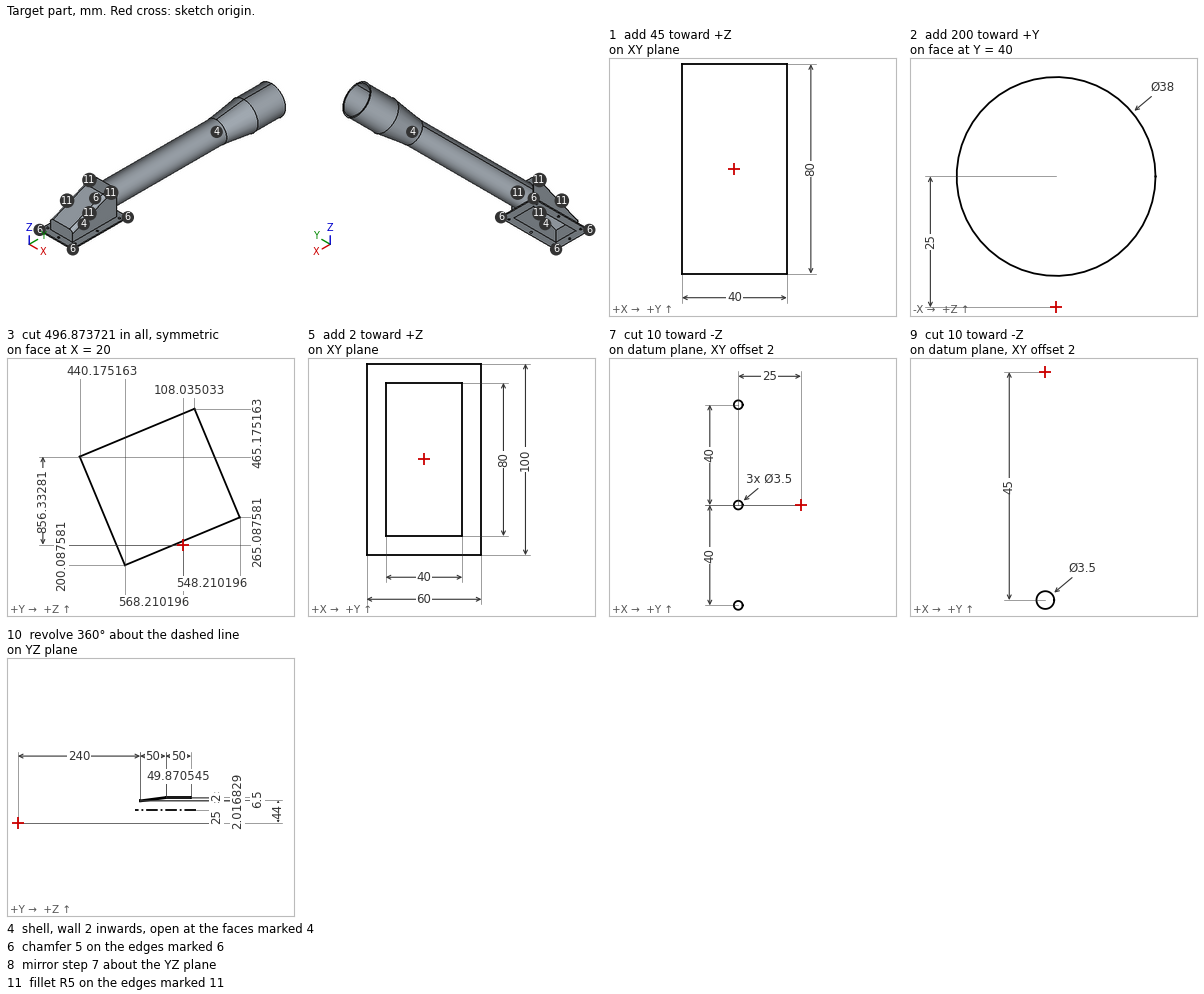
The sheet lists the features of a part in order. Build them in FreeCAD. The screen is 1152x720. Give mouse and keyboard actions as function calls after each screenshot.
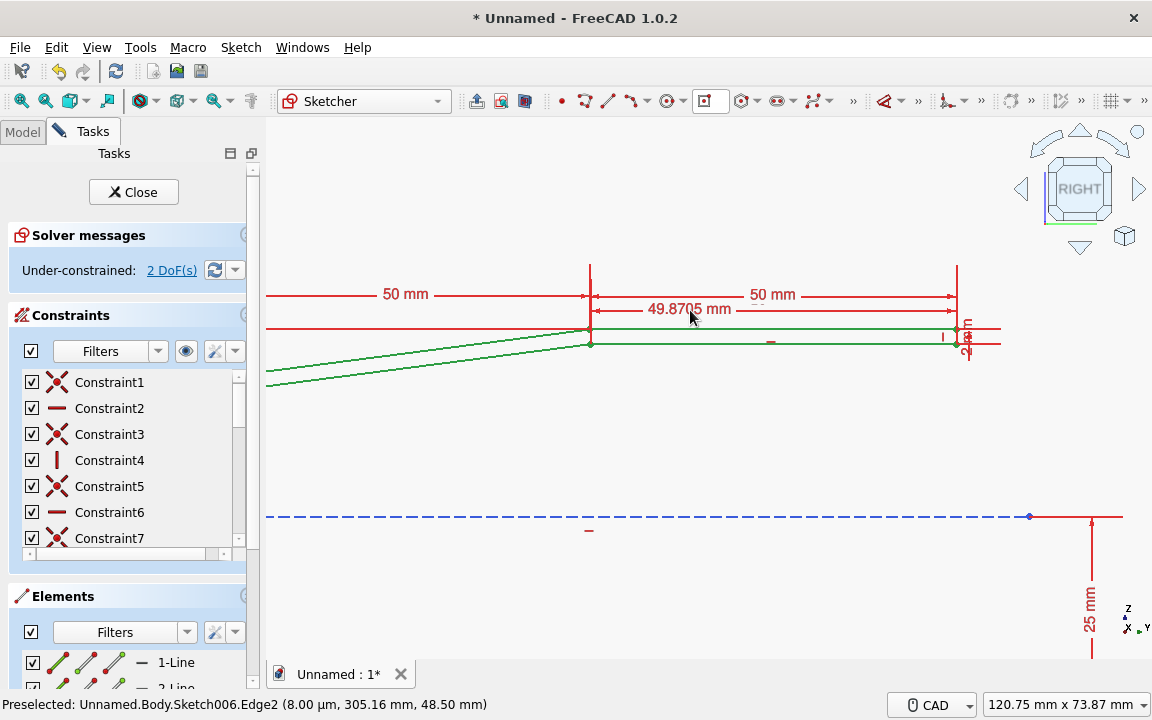
click(134, 192)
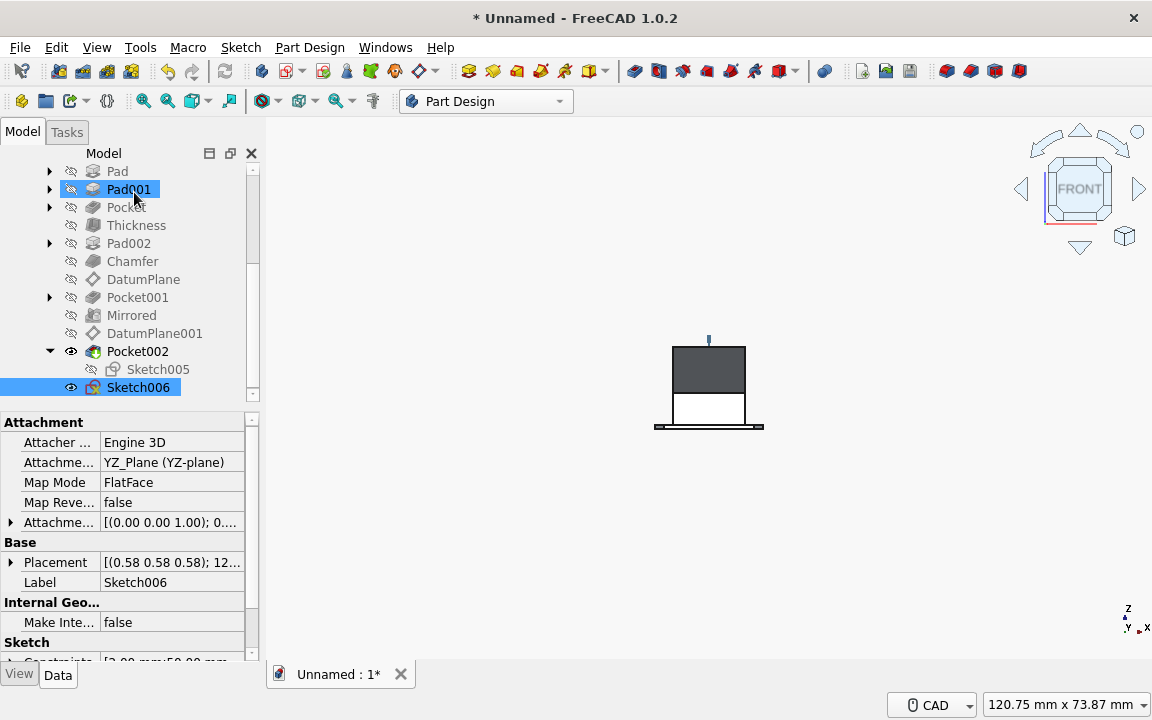
click(494, 72)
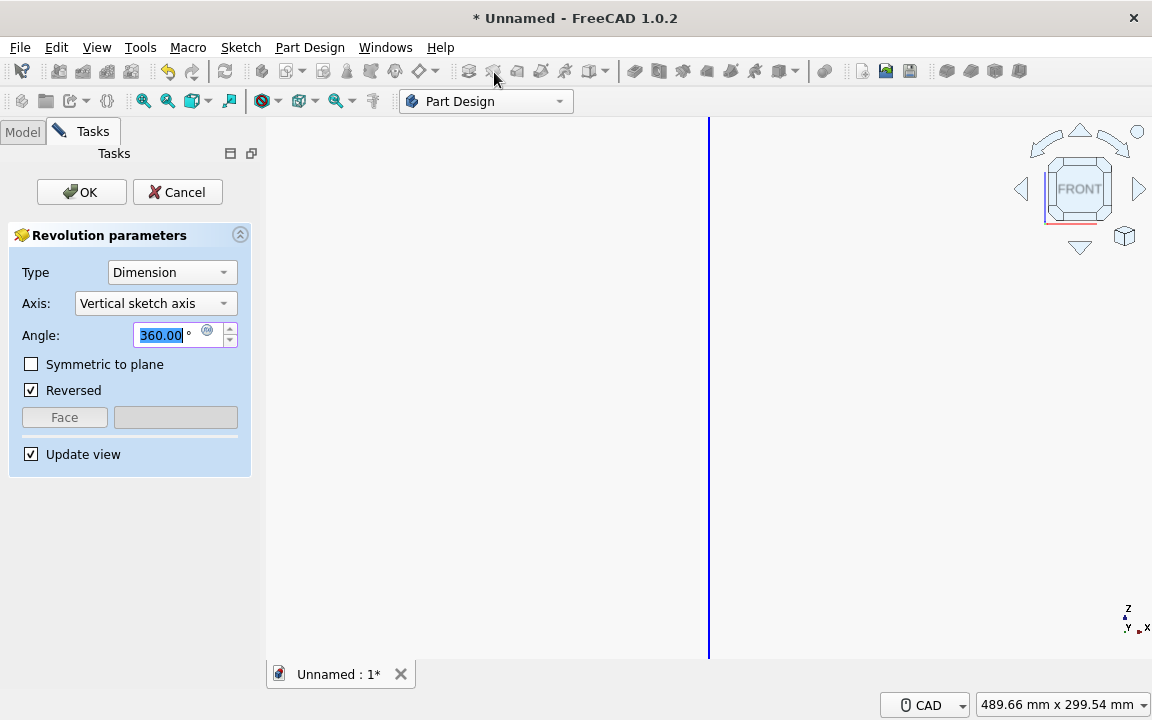
click(156, 304)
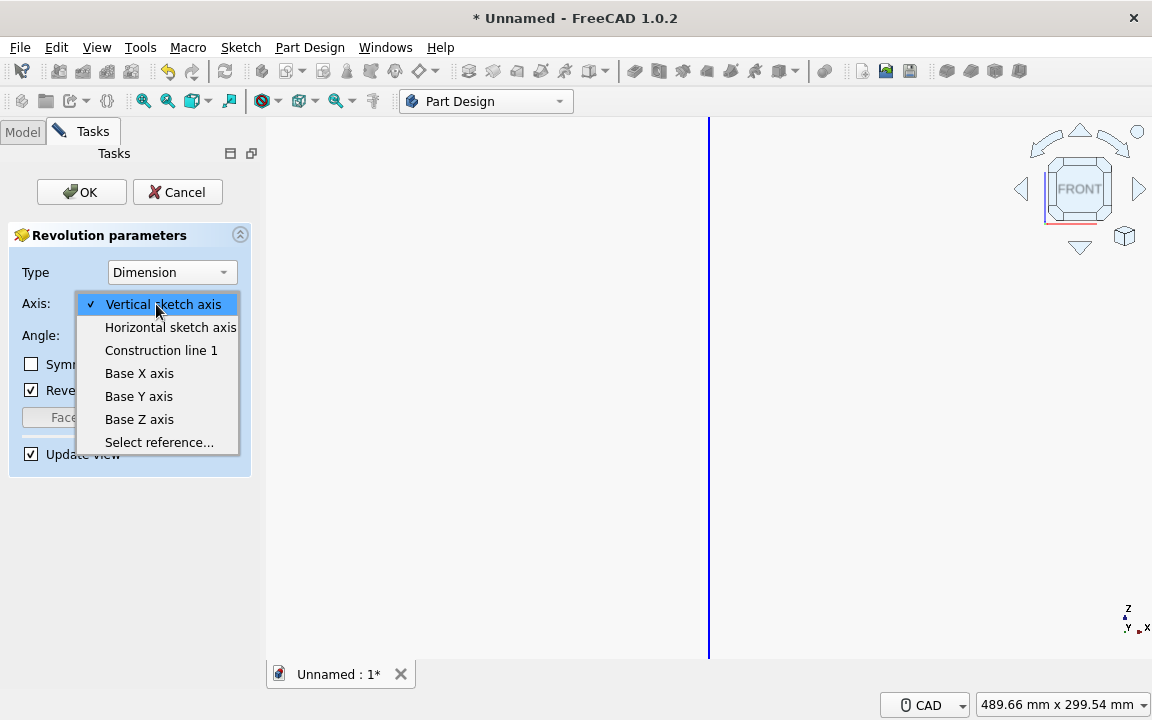
click(156, 350)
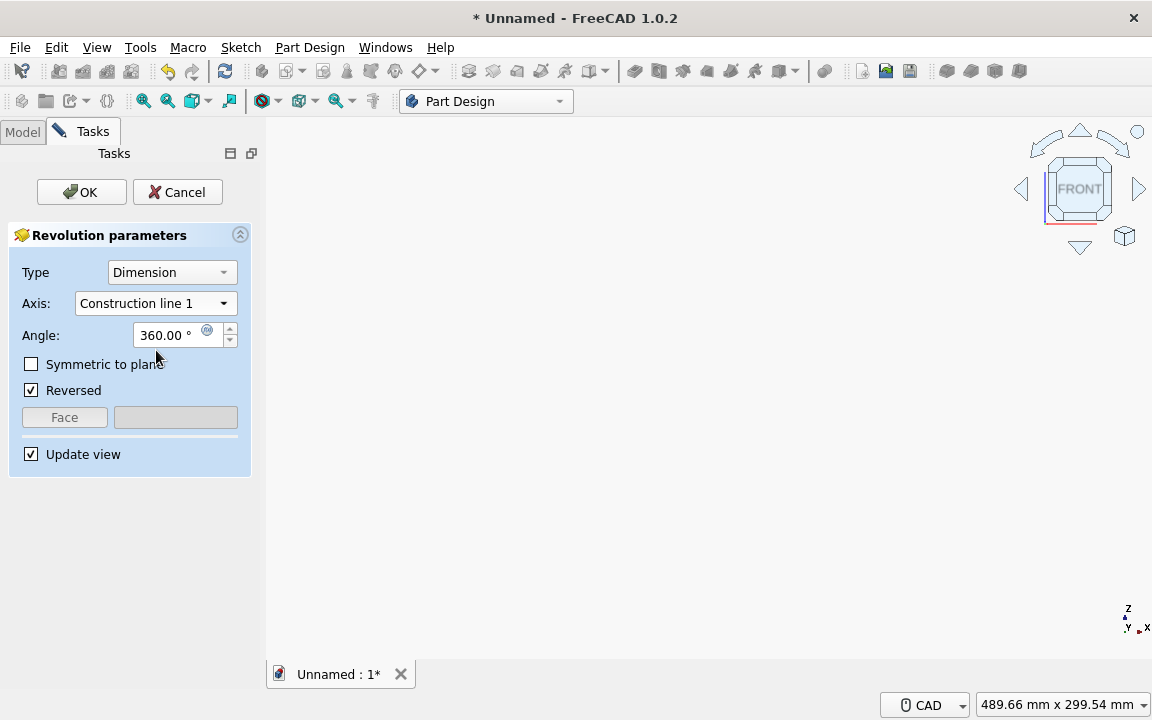
click(82, 192)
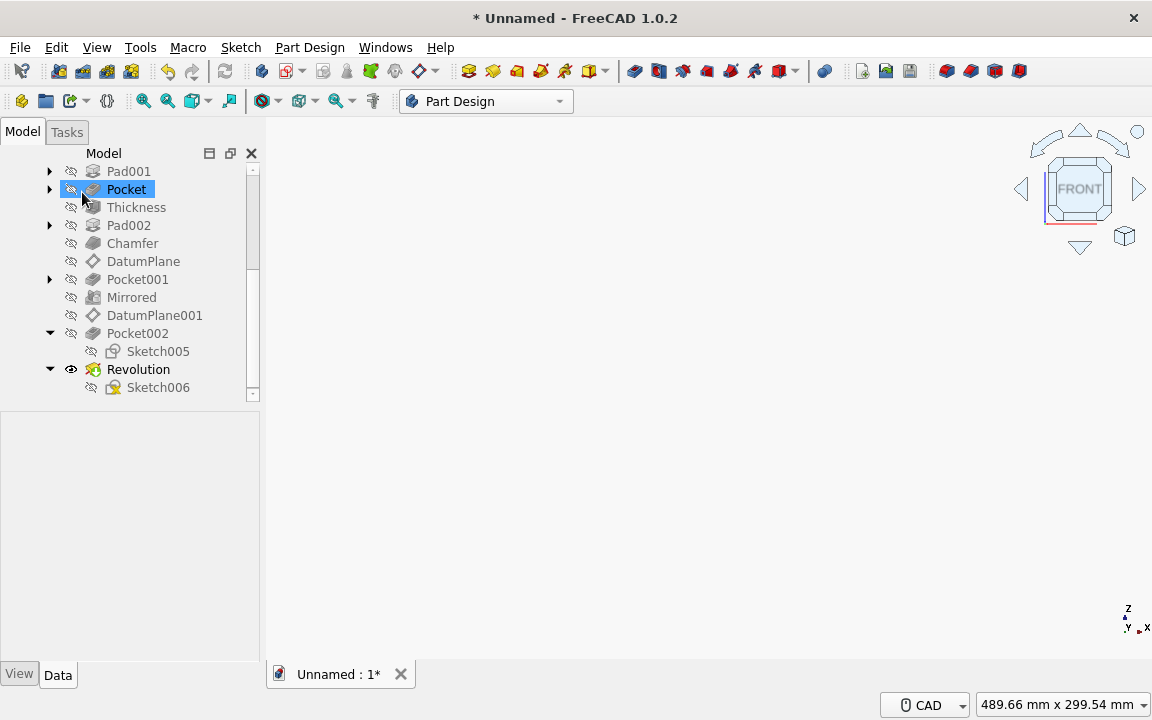
key(v)
key(f)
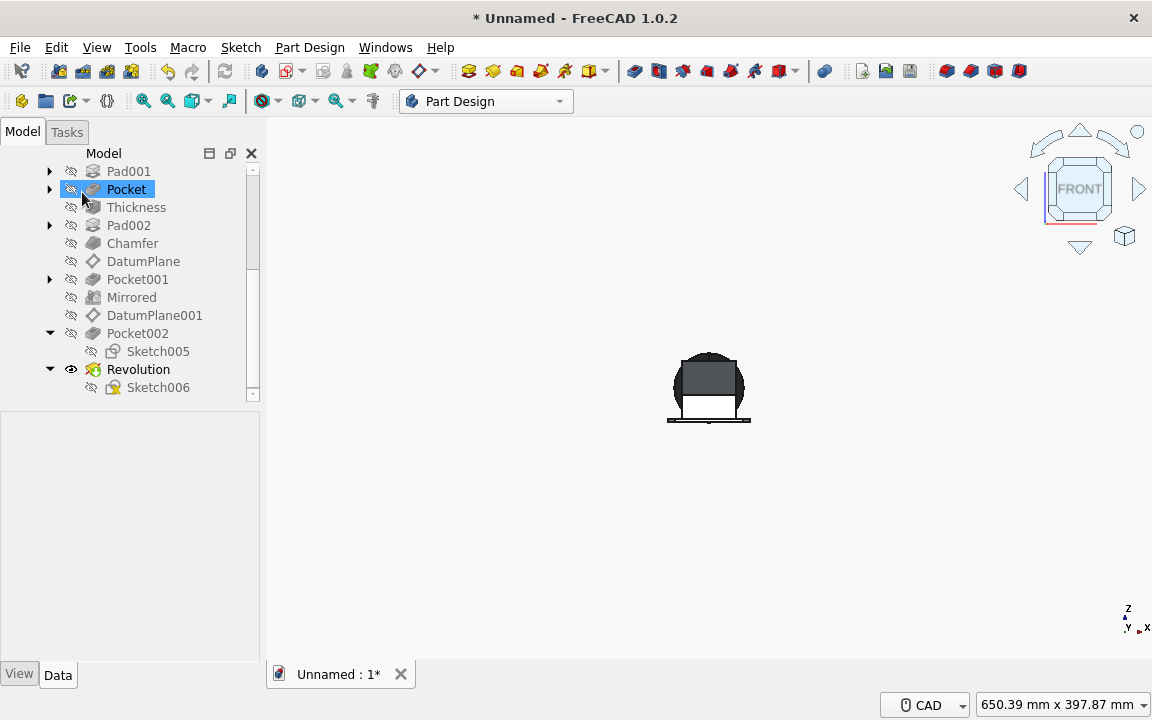
click(736, 377)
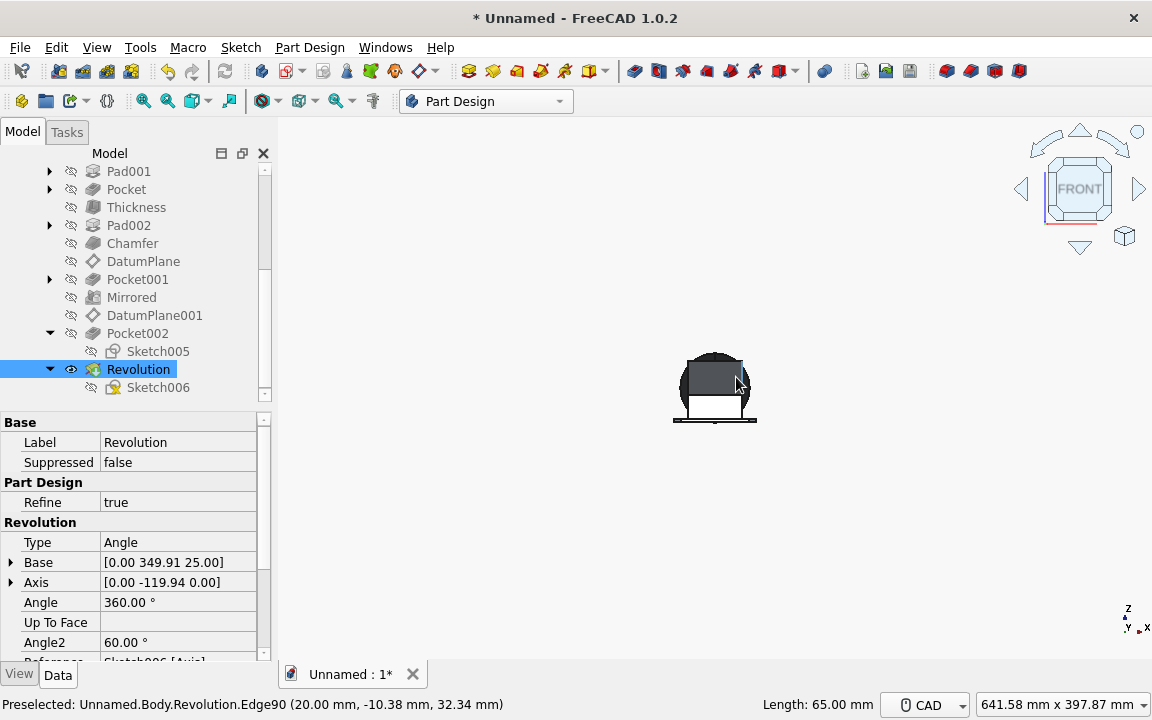
click(688, 377, ctrl)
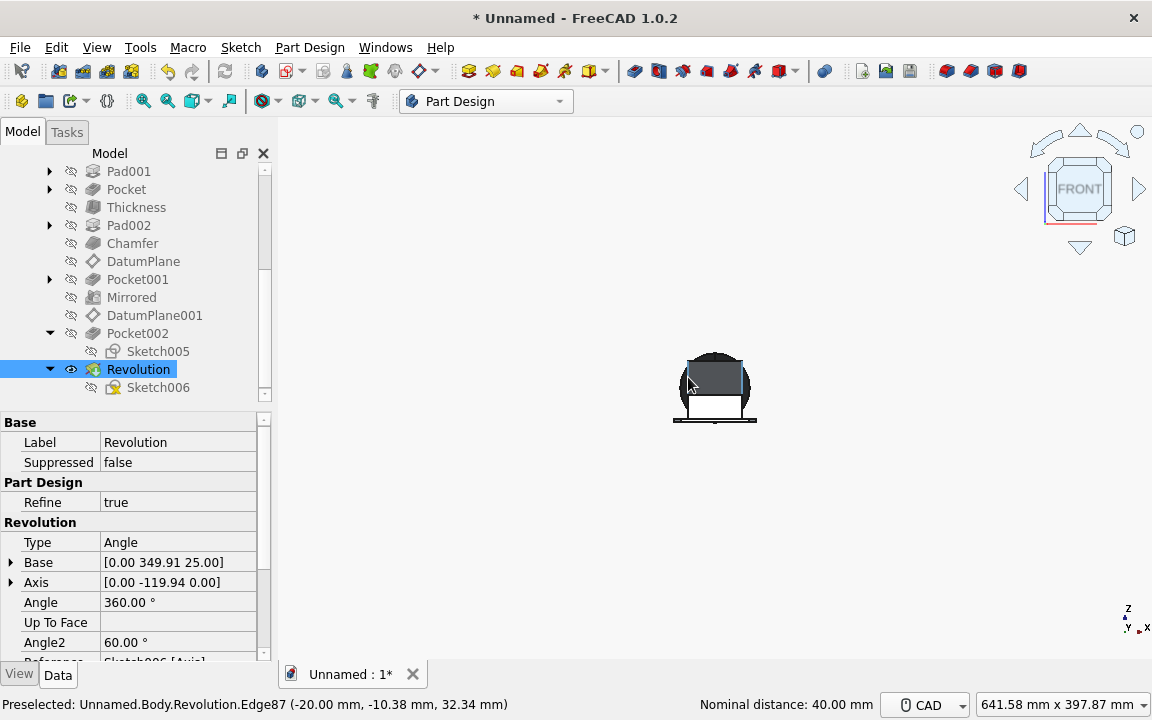
key(0)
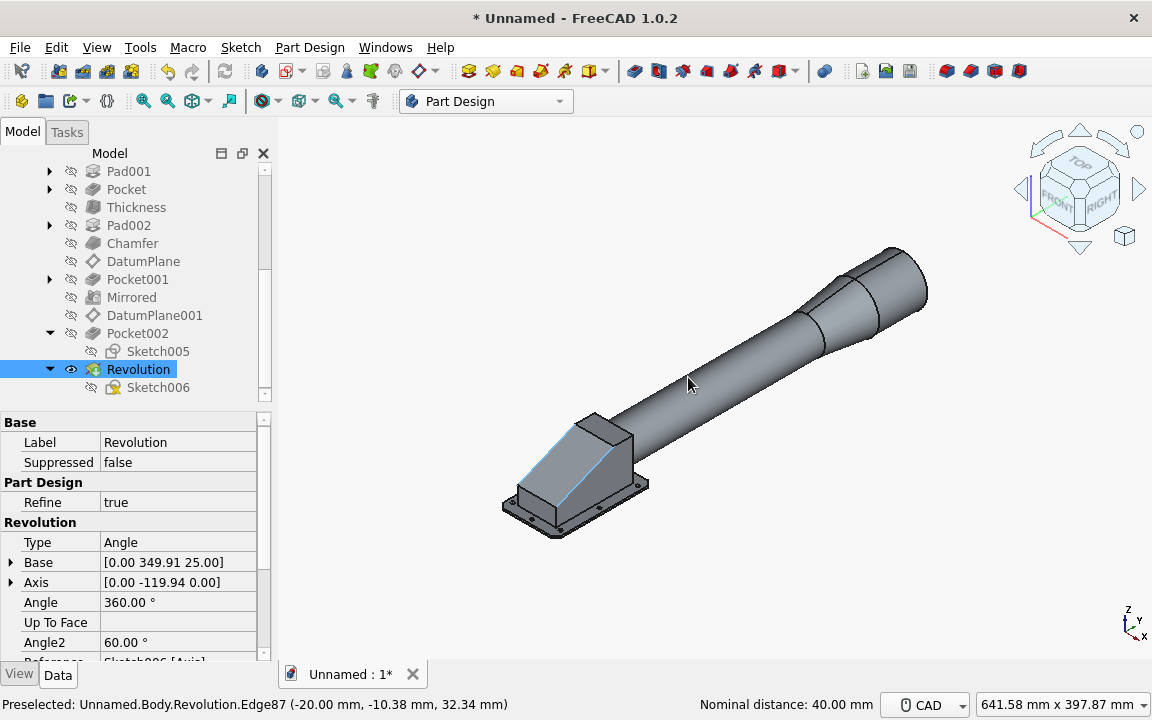
click(623, 440, ctrl)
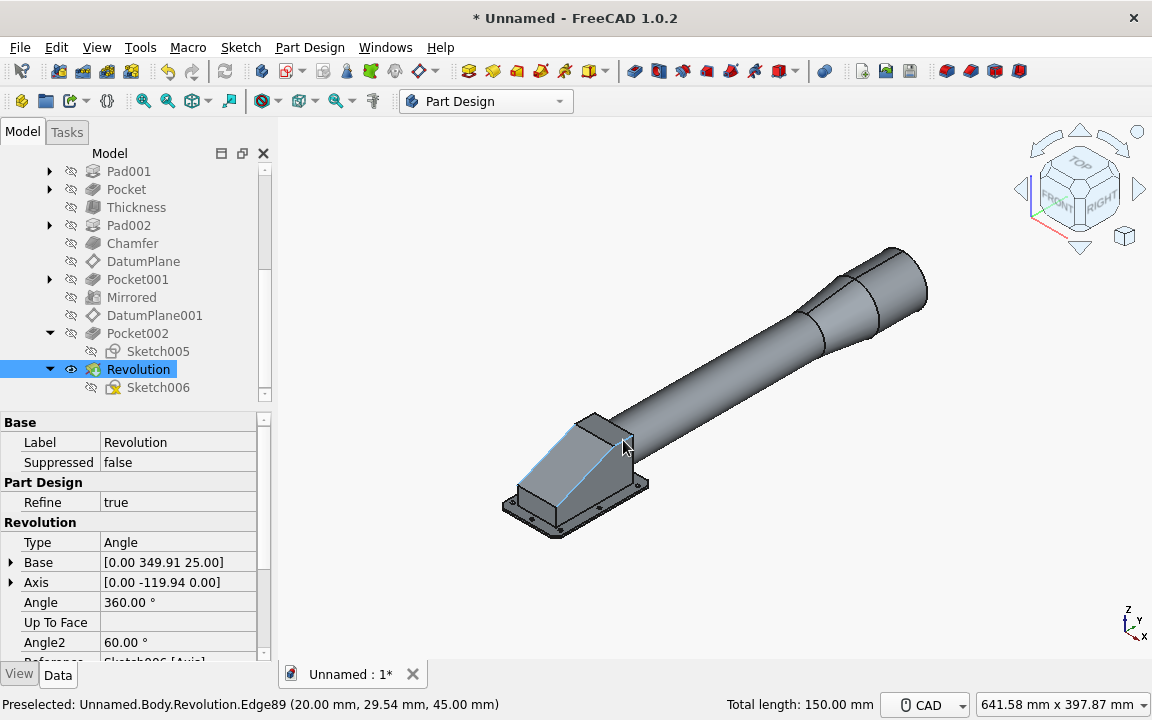
key(2)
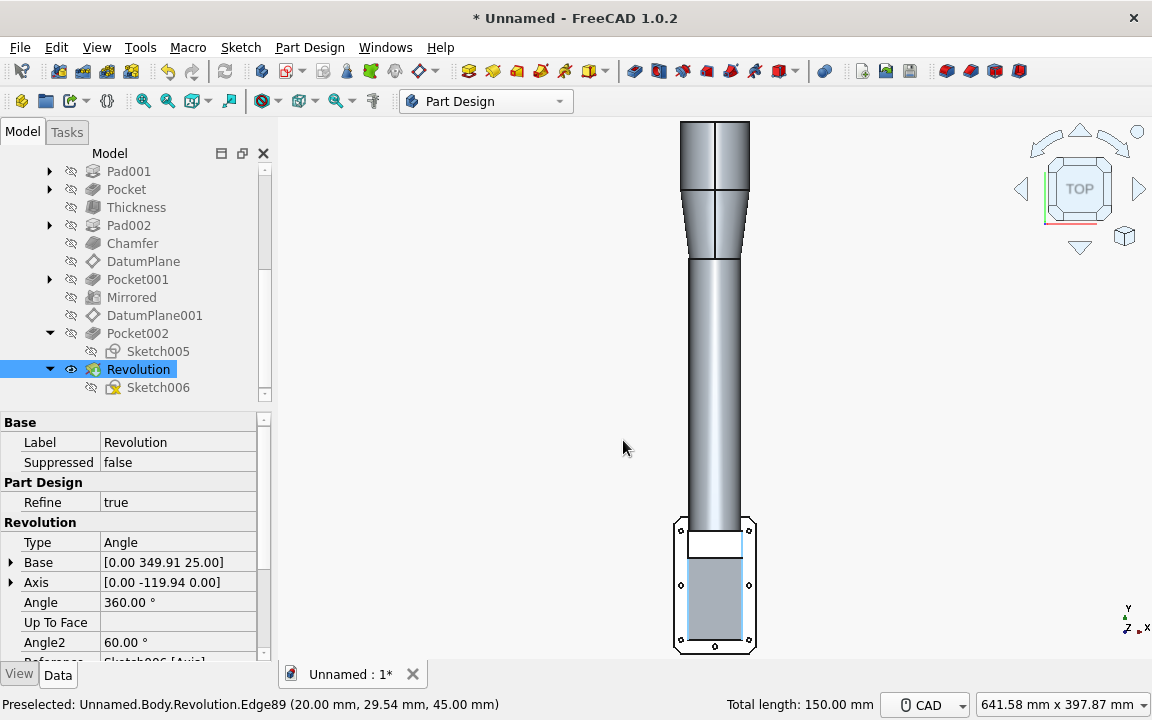
click(688, 544, ctrl)